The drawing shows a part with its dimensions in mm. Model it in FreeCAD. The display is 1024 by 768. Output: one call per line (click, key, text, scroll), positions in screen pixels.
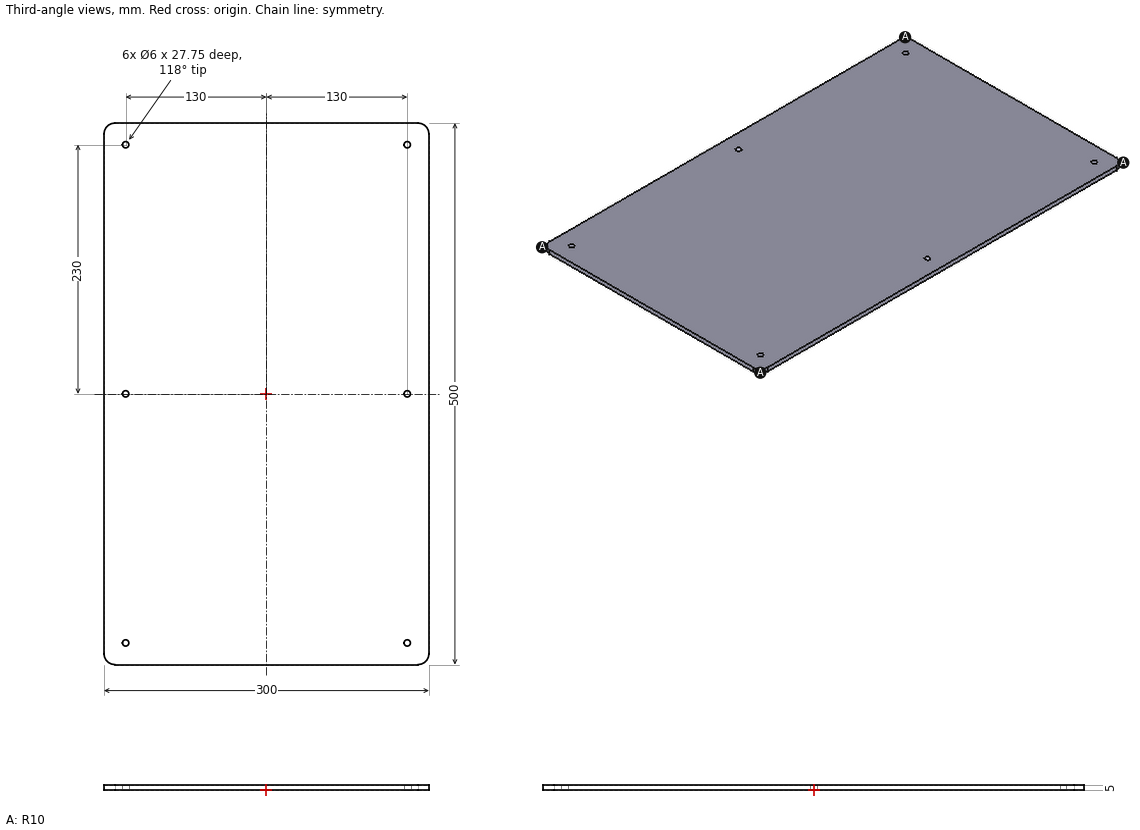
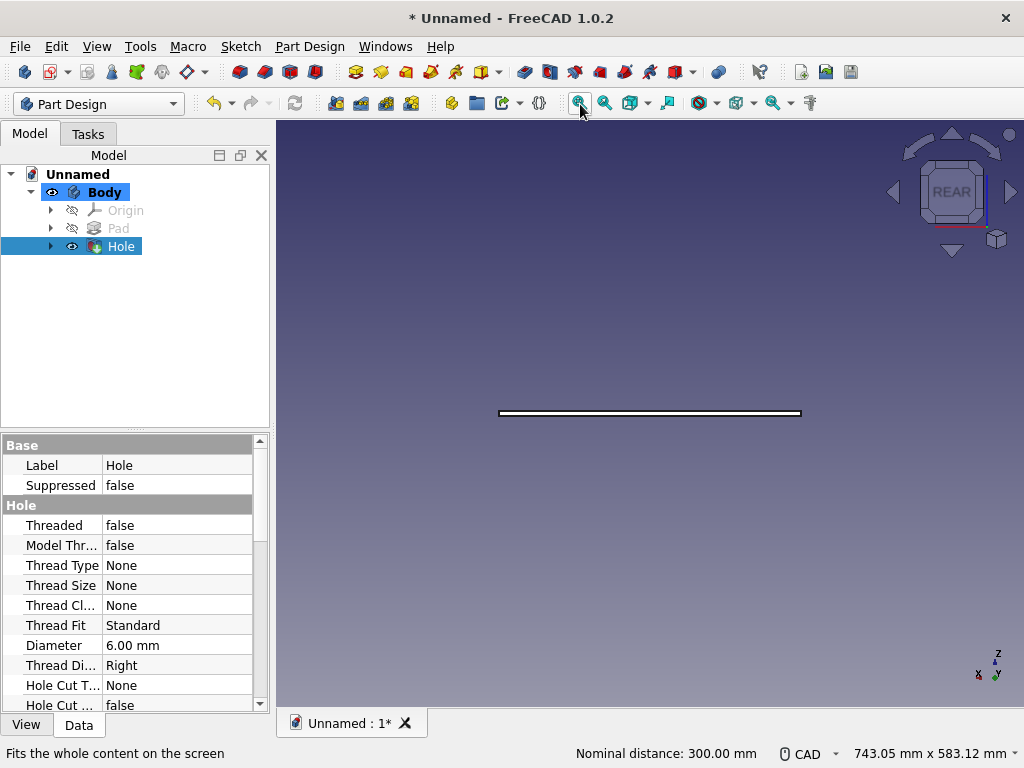
click(580, 104)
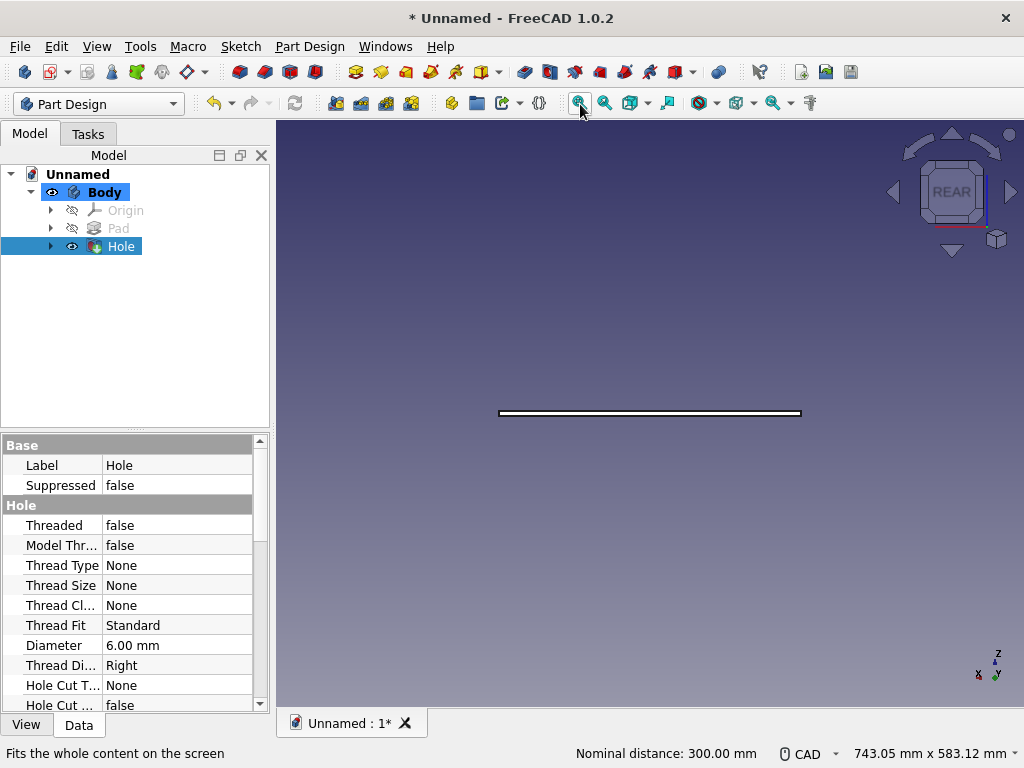
scroll(801, 413, up, 11)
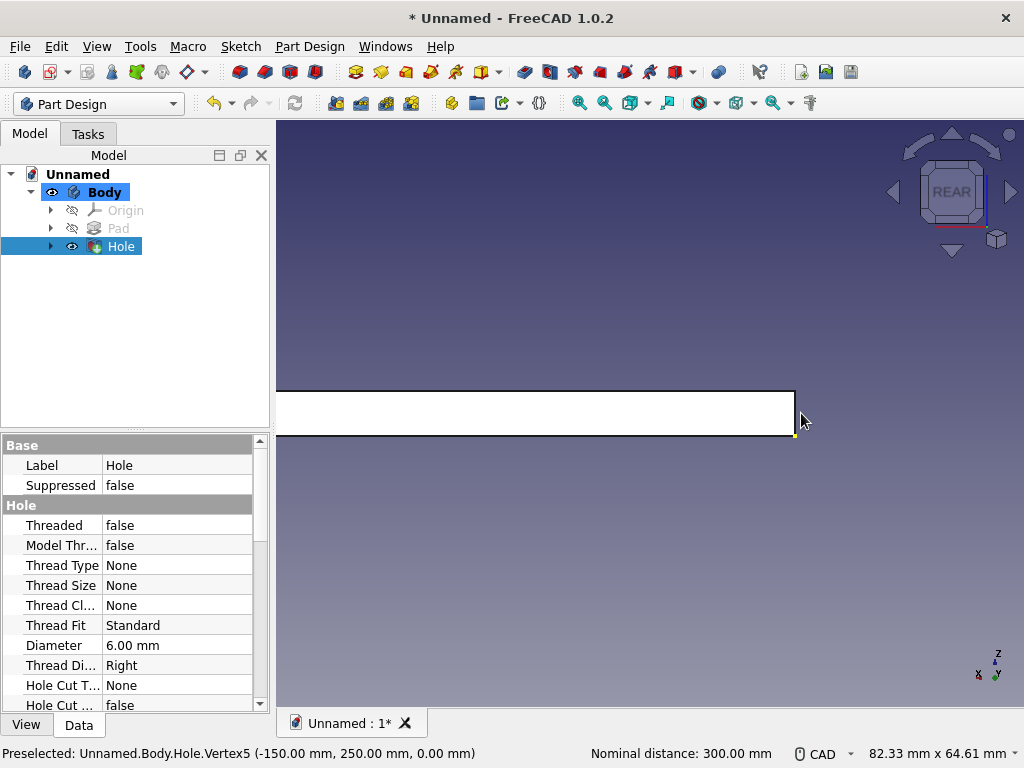
click(795, 413, ctrl)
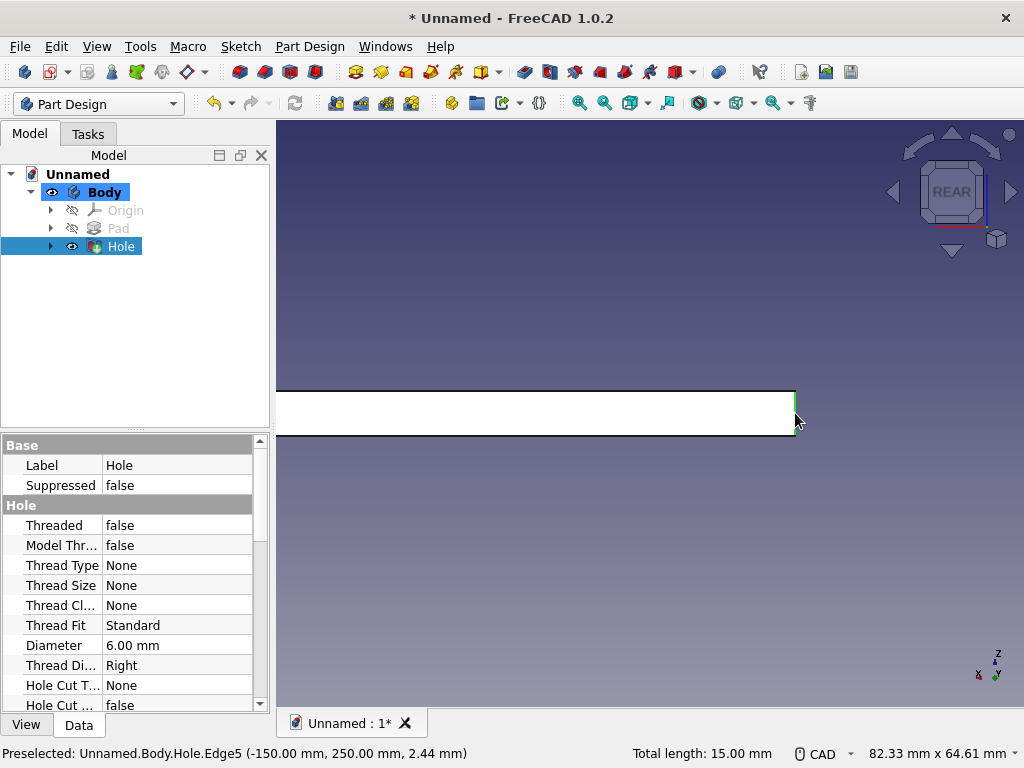
click(580, 104)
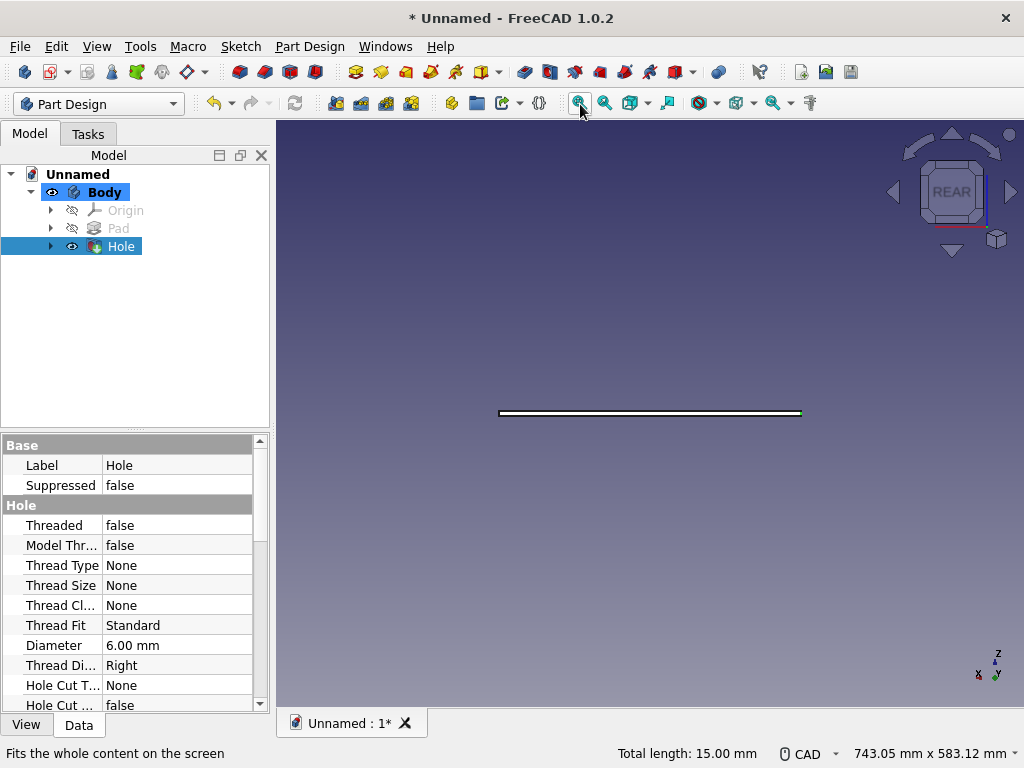
key(6)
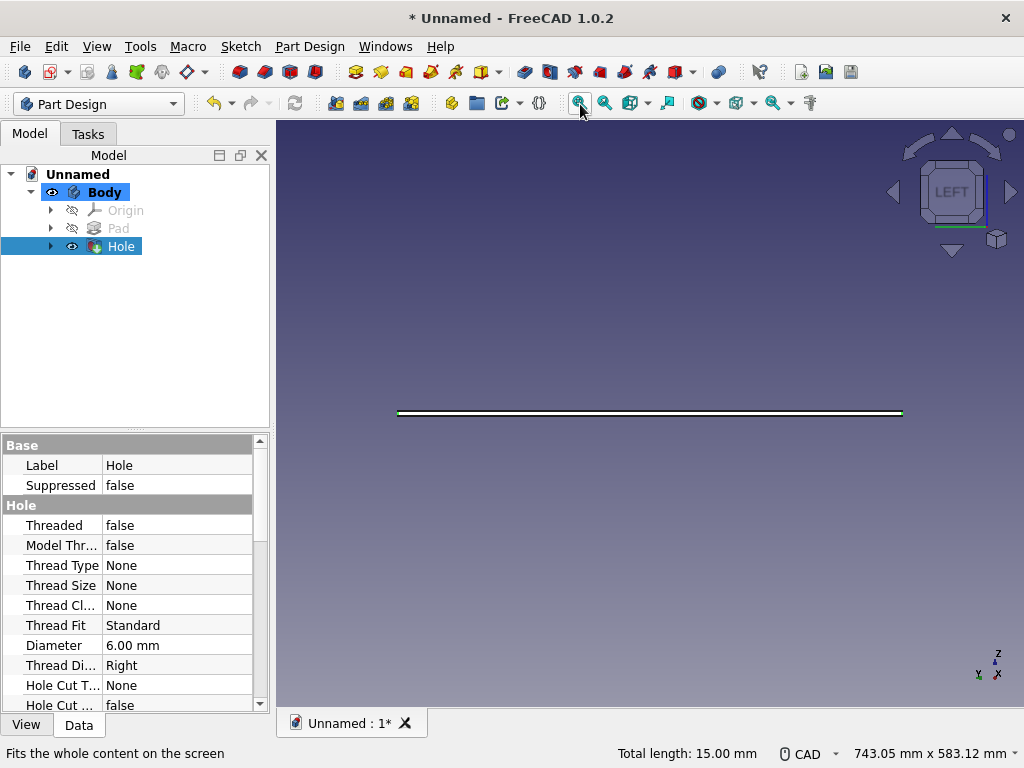
scroll(398, 412, up, 11)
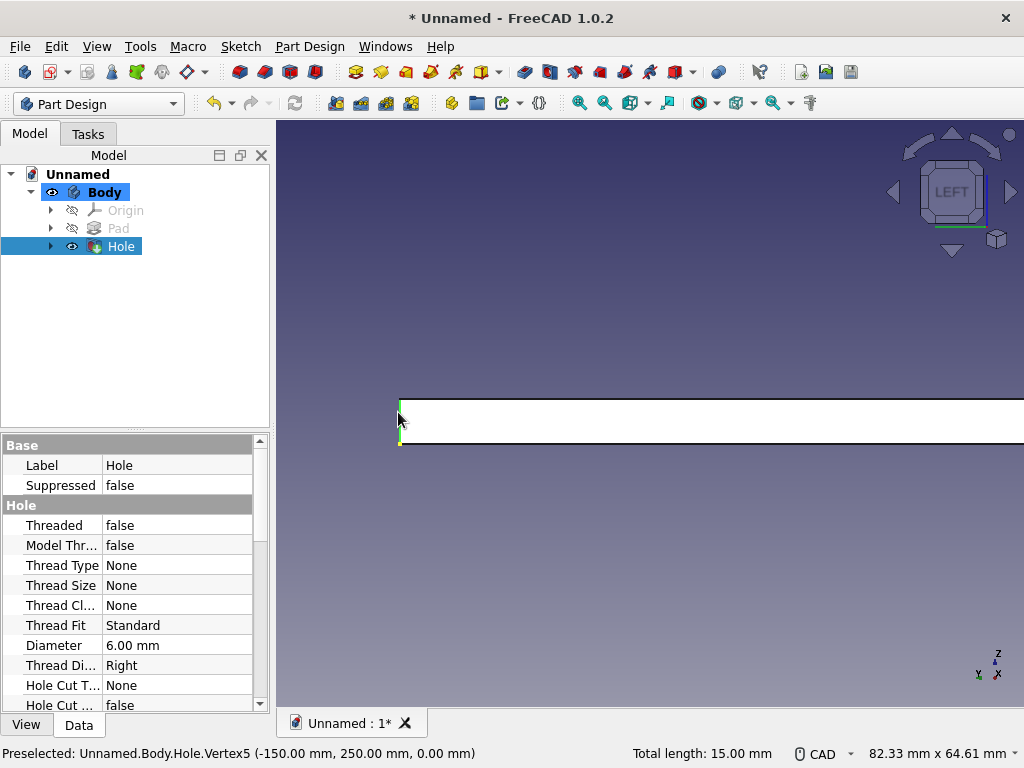
click(580, 104)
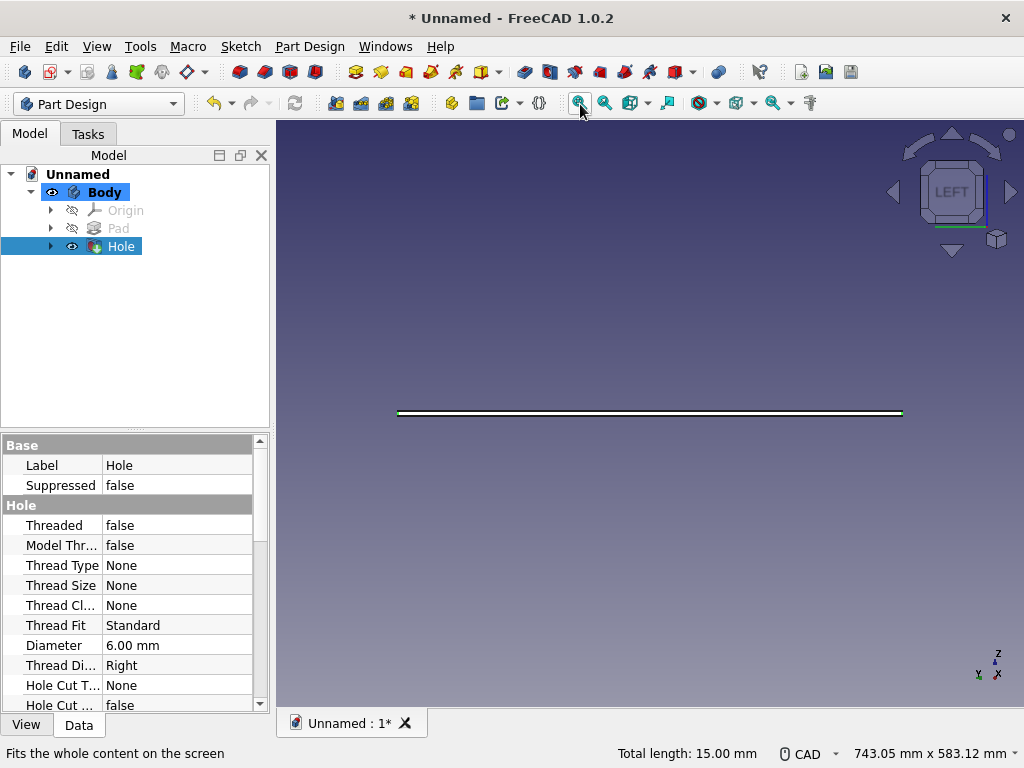
key(v)
key(3)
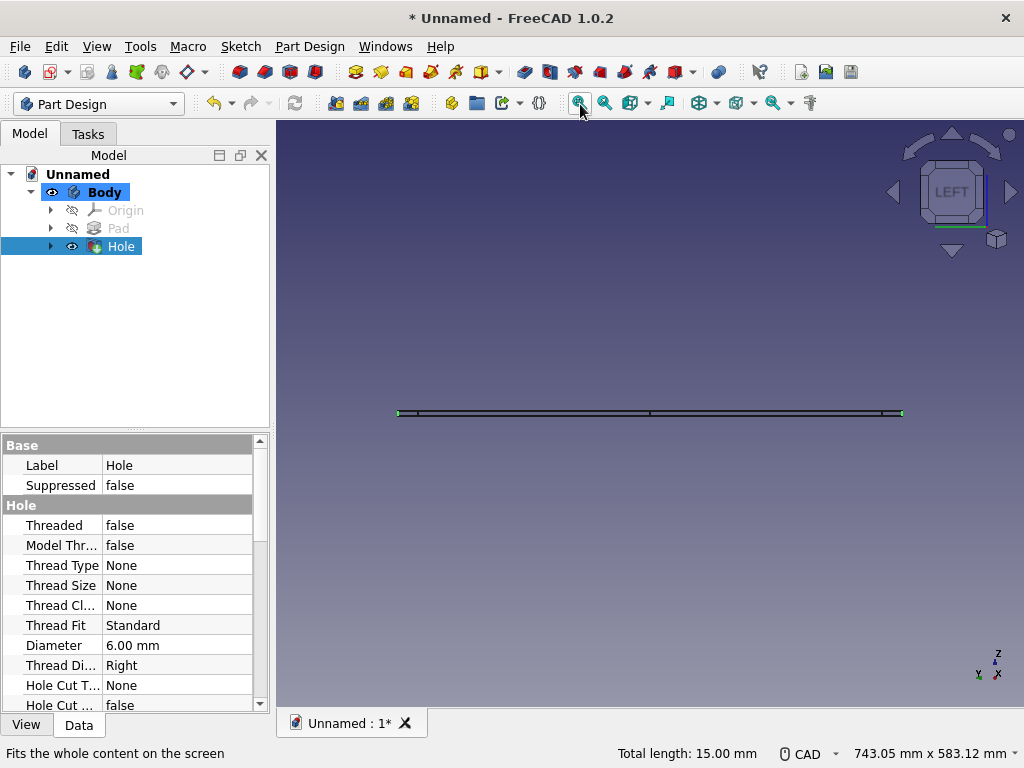
key(0)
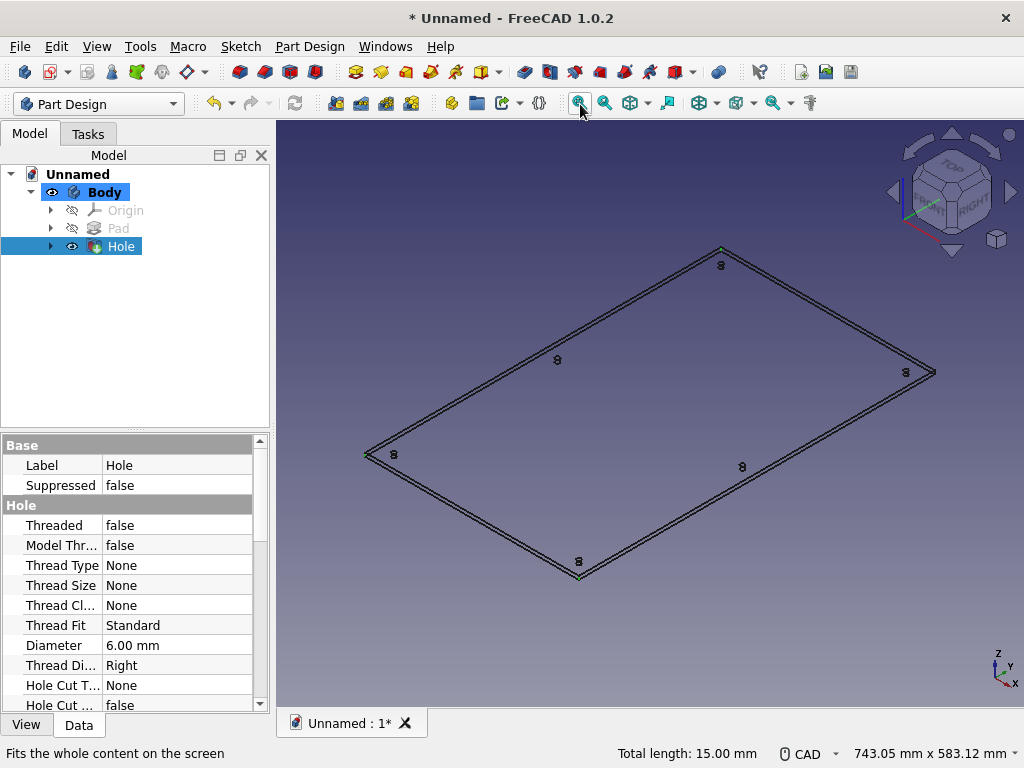
key(2)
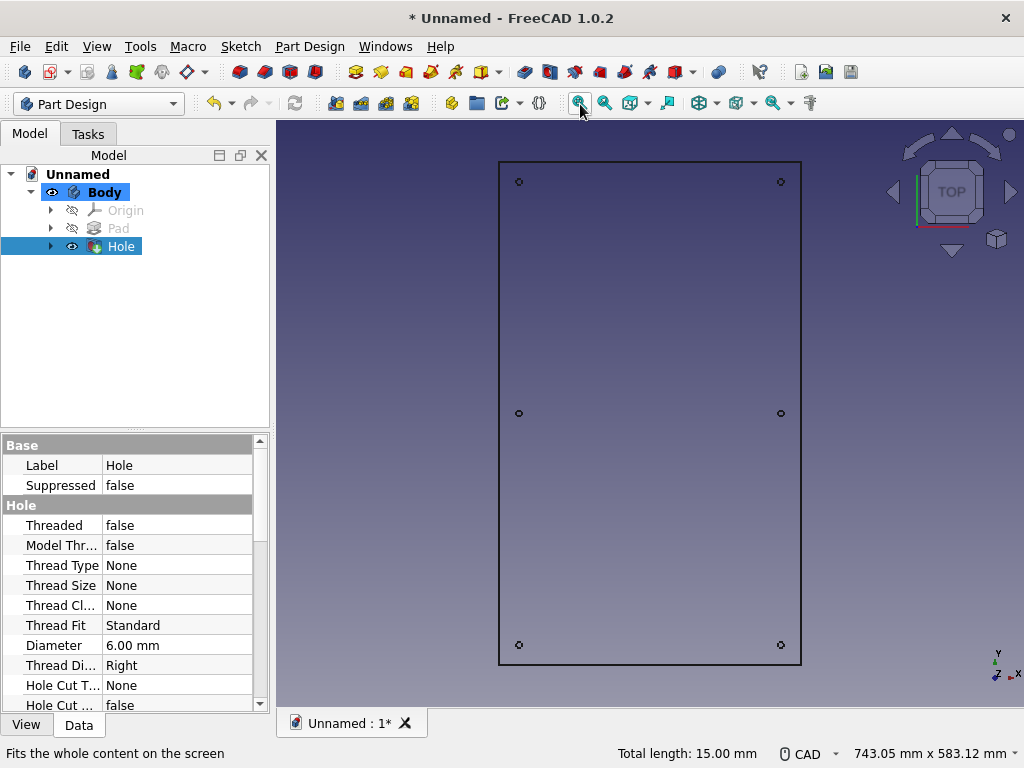
scroll(801, 161, up, 11)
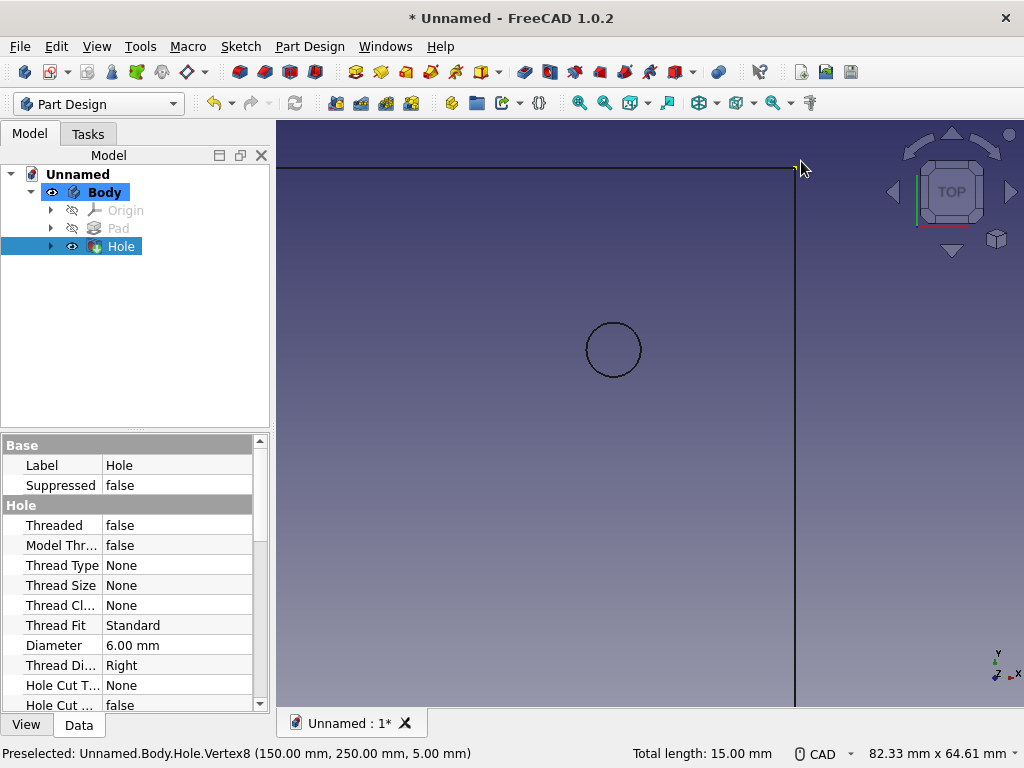
click(580, 104)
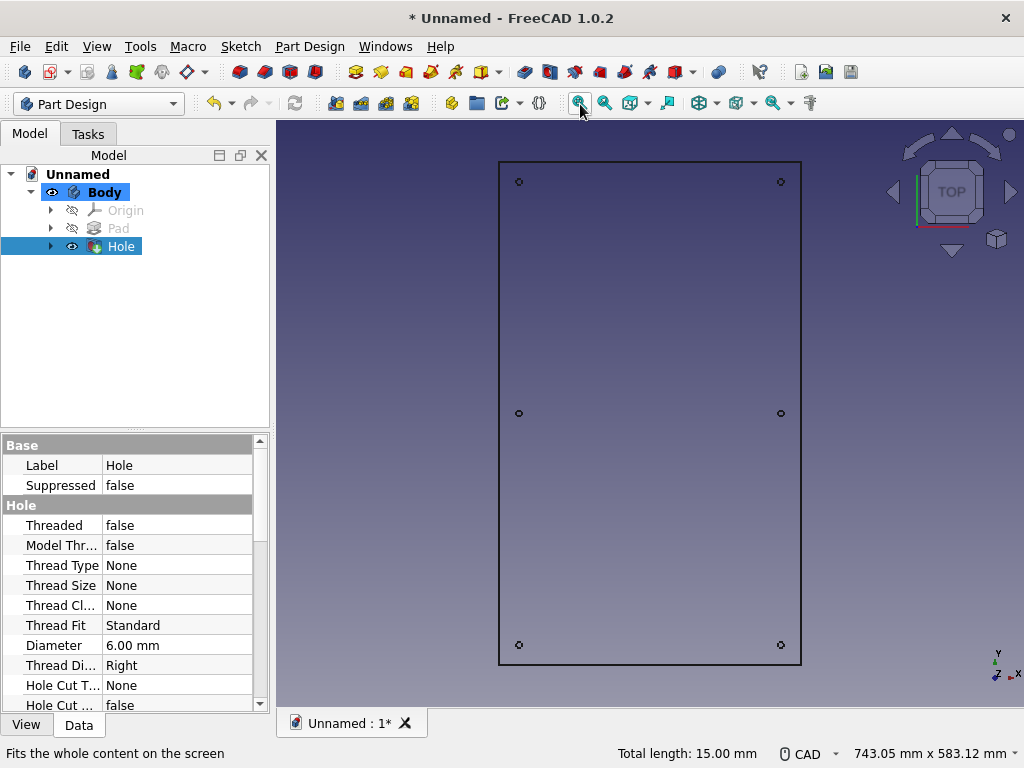
key(1)